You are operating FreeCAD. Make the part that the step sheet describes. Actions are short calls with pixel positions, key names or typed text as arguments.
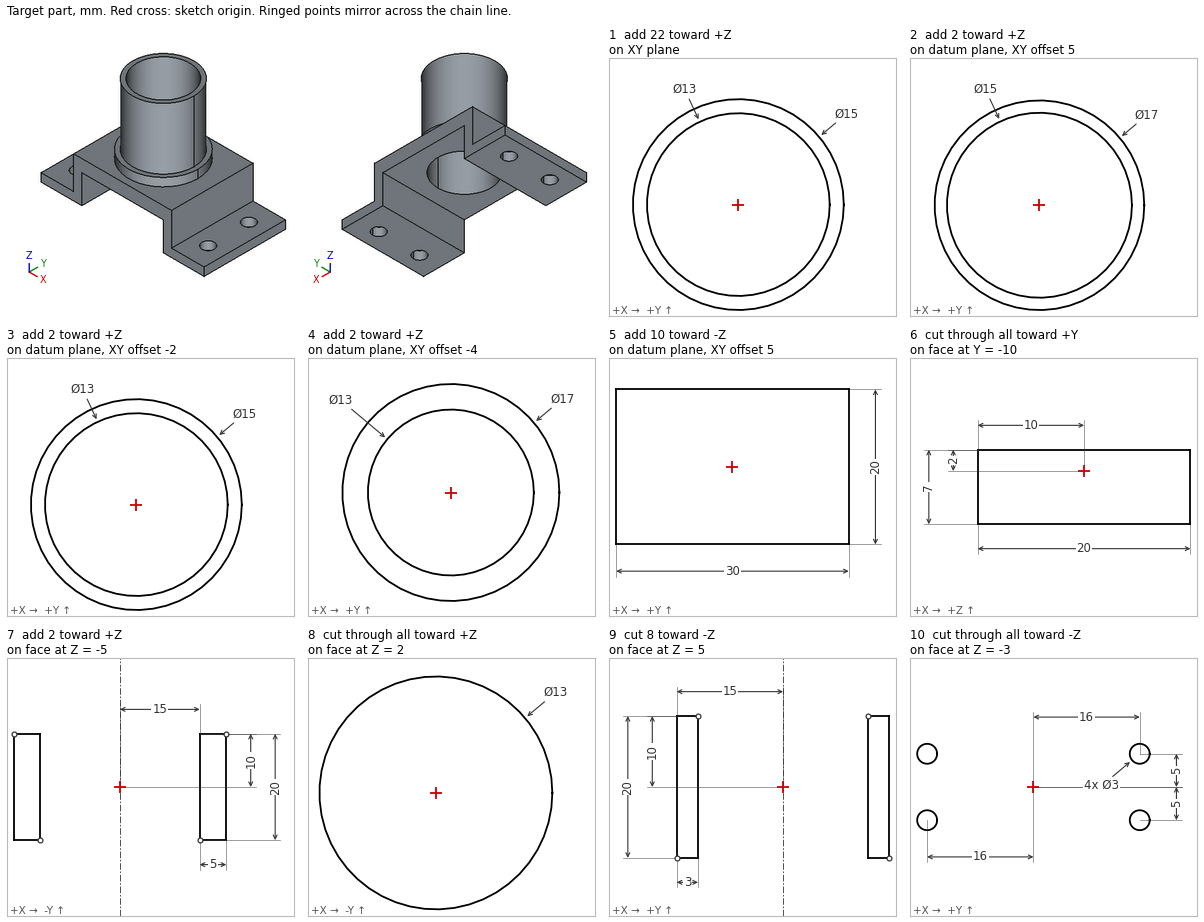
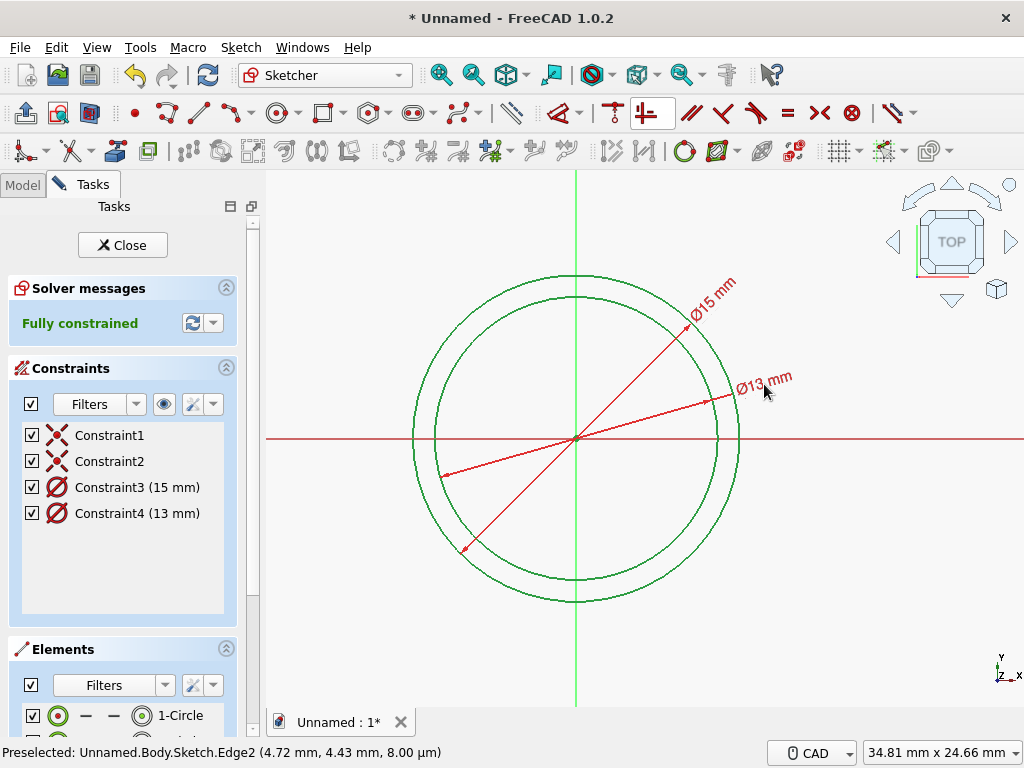
click(123, 245)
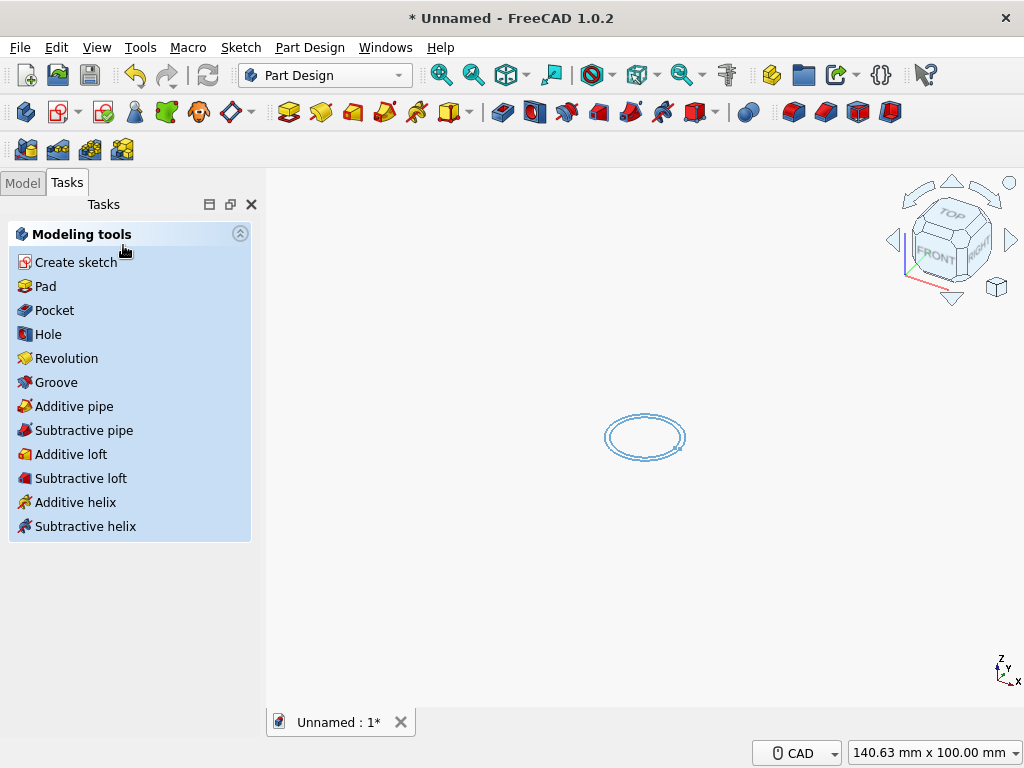
click(290, 112)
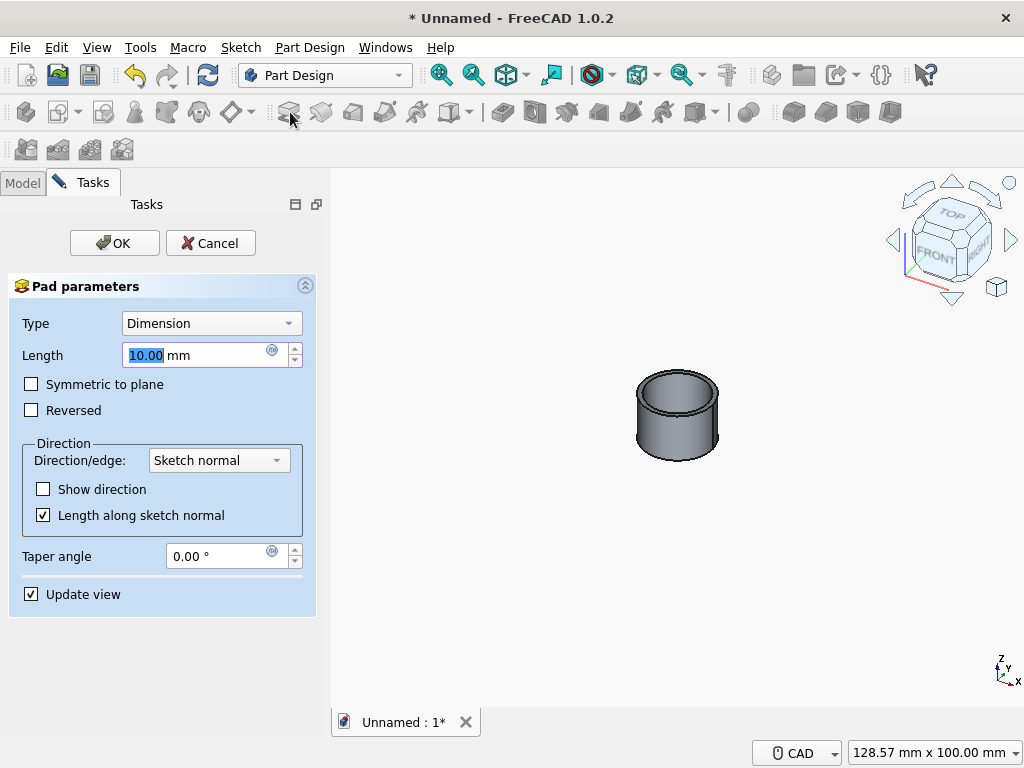
text(22)
key(Tab)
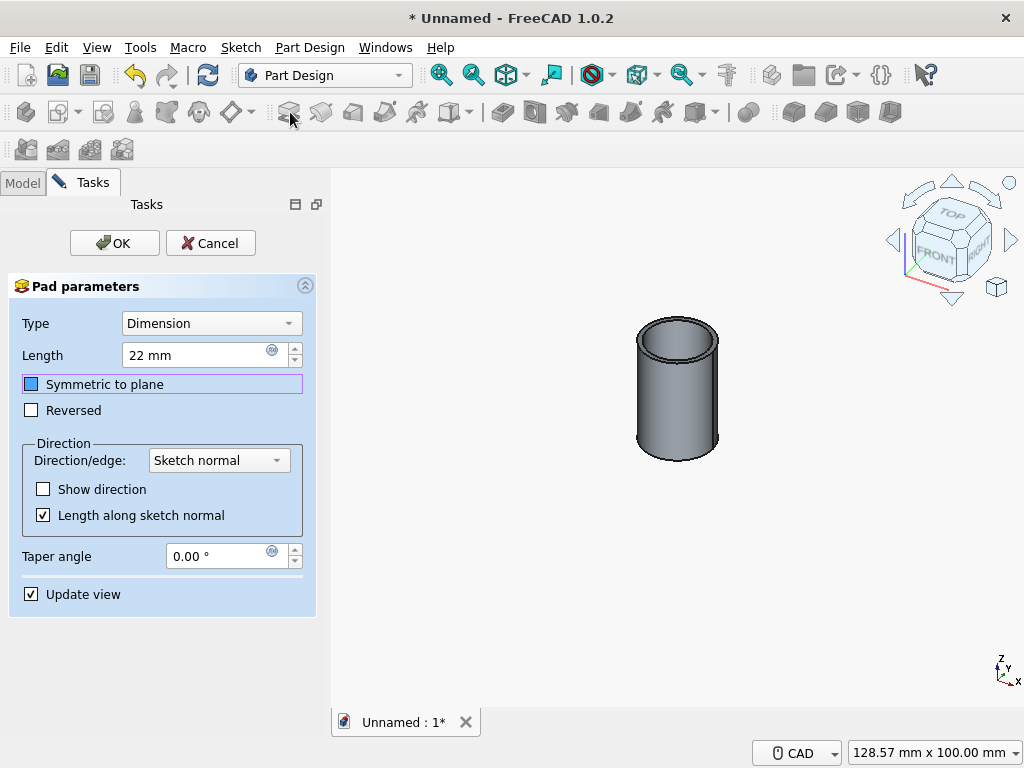
click(115, 243)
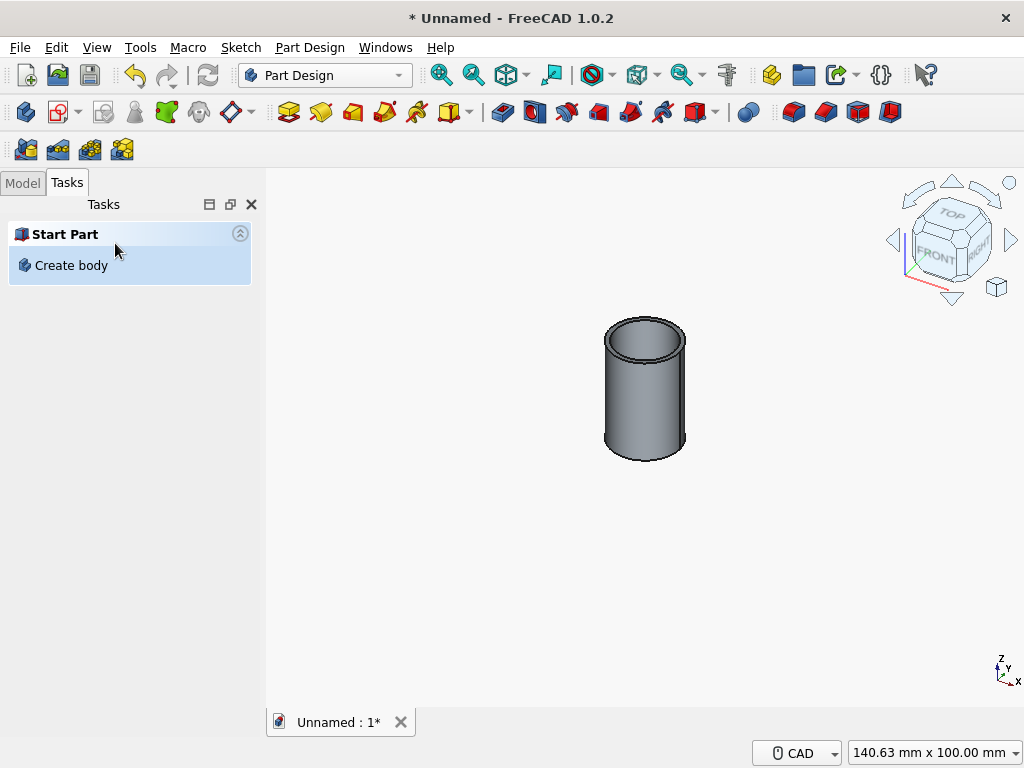
click(442, 76)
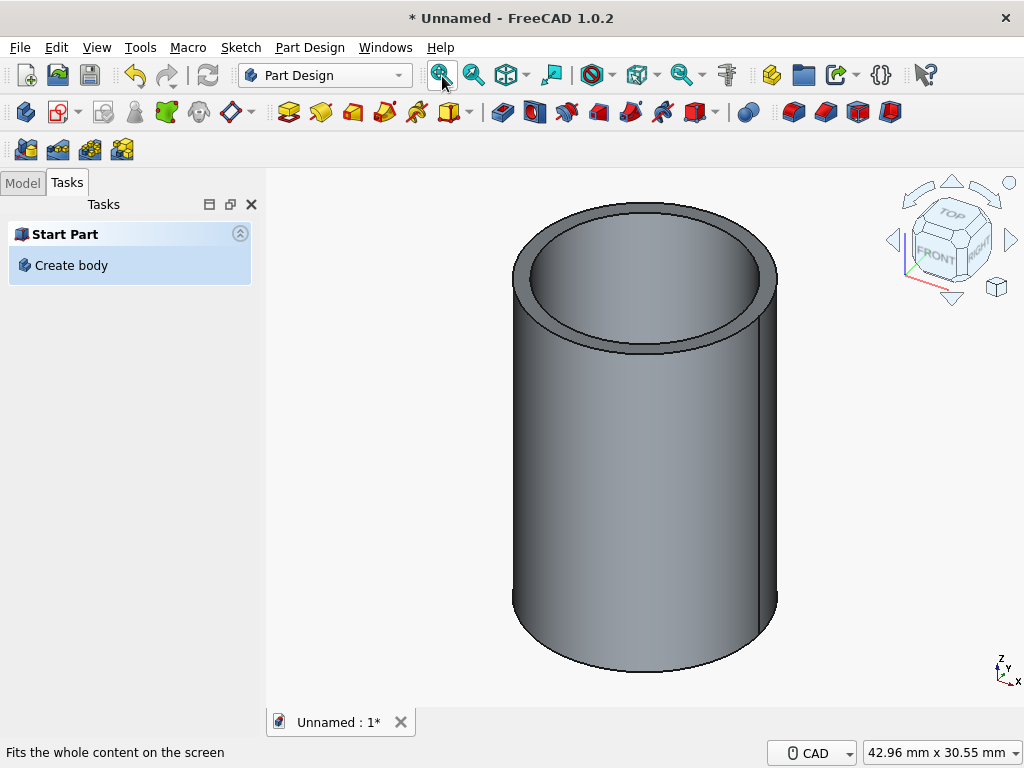
click(23, 182)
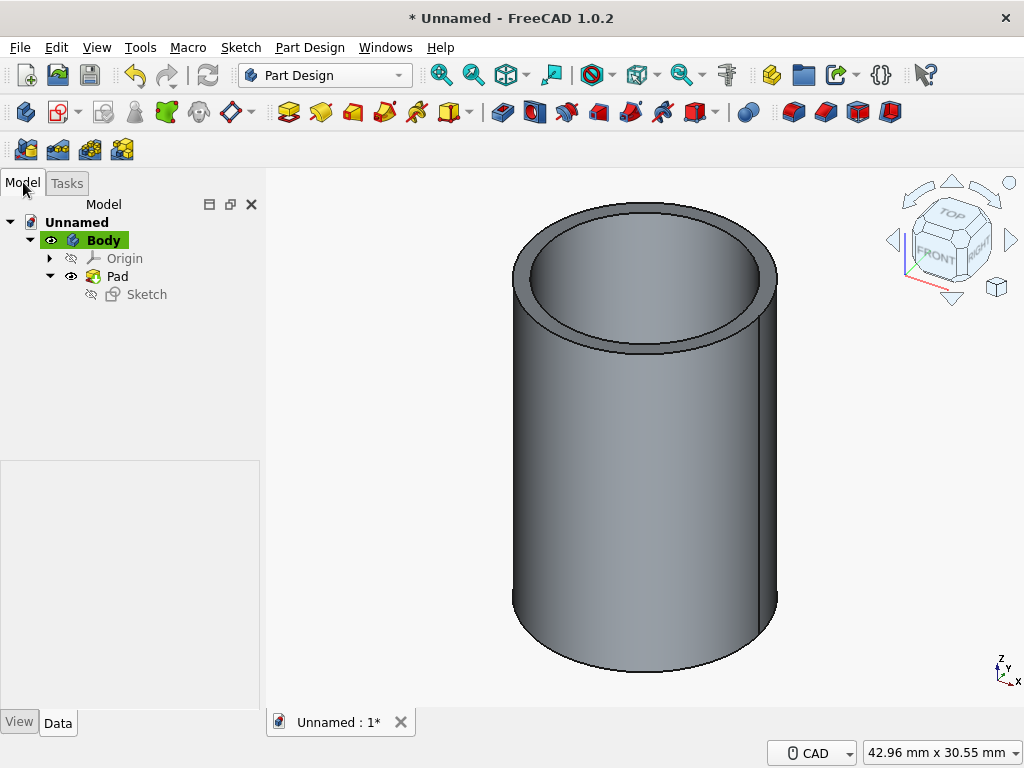
click(50, 258)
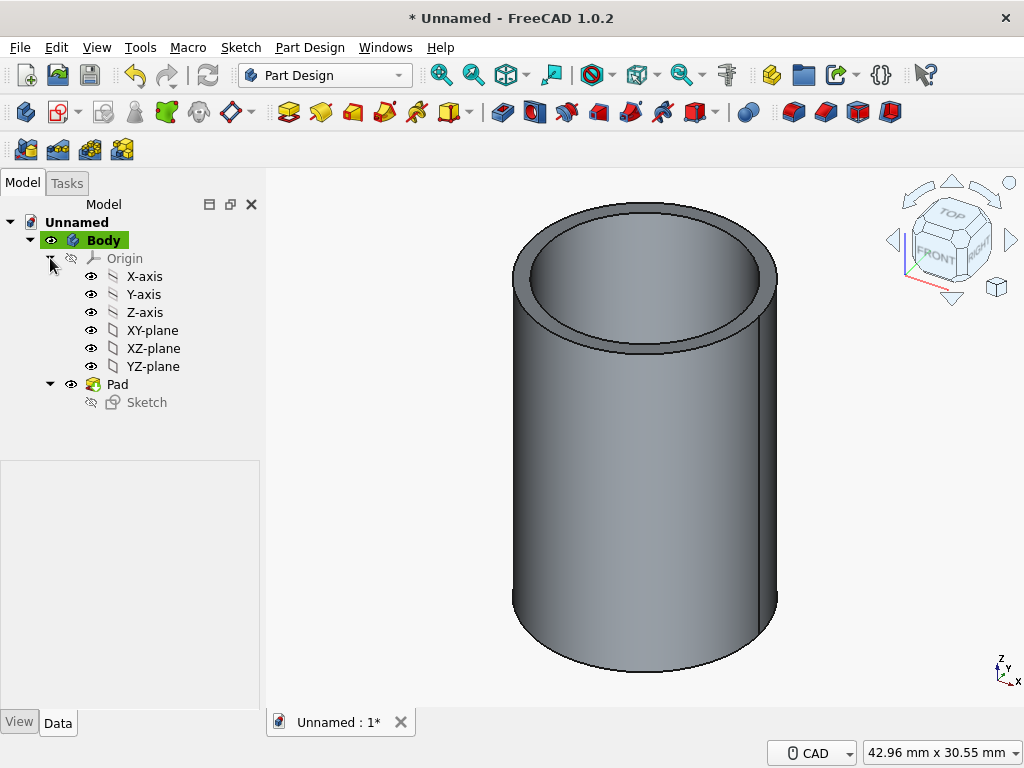
click(136, 330)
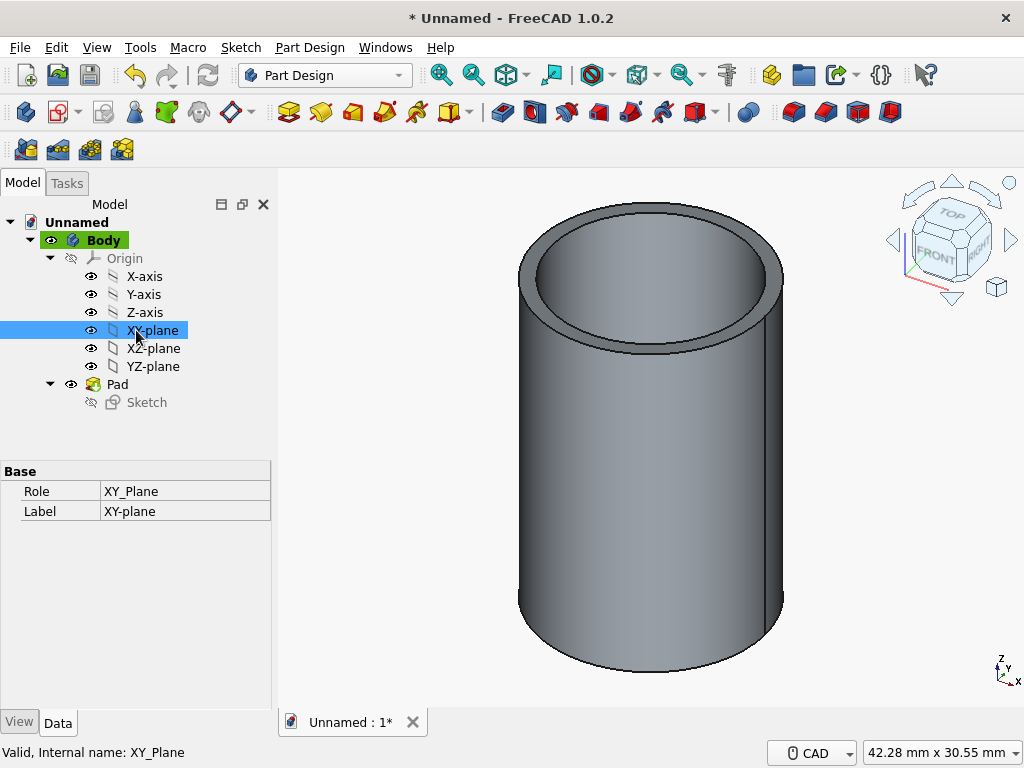
click(232, 112)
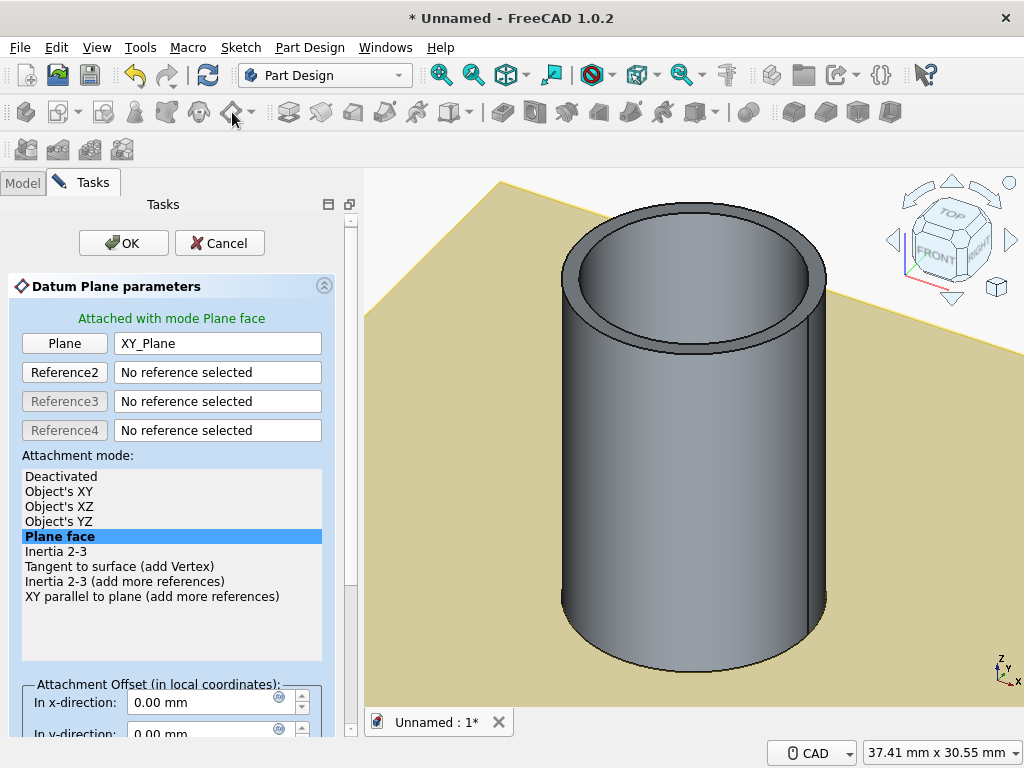
scroll(351, 475, down, 2)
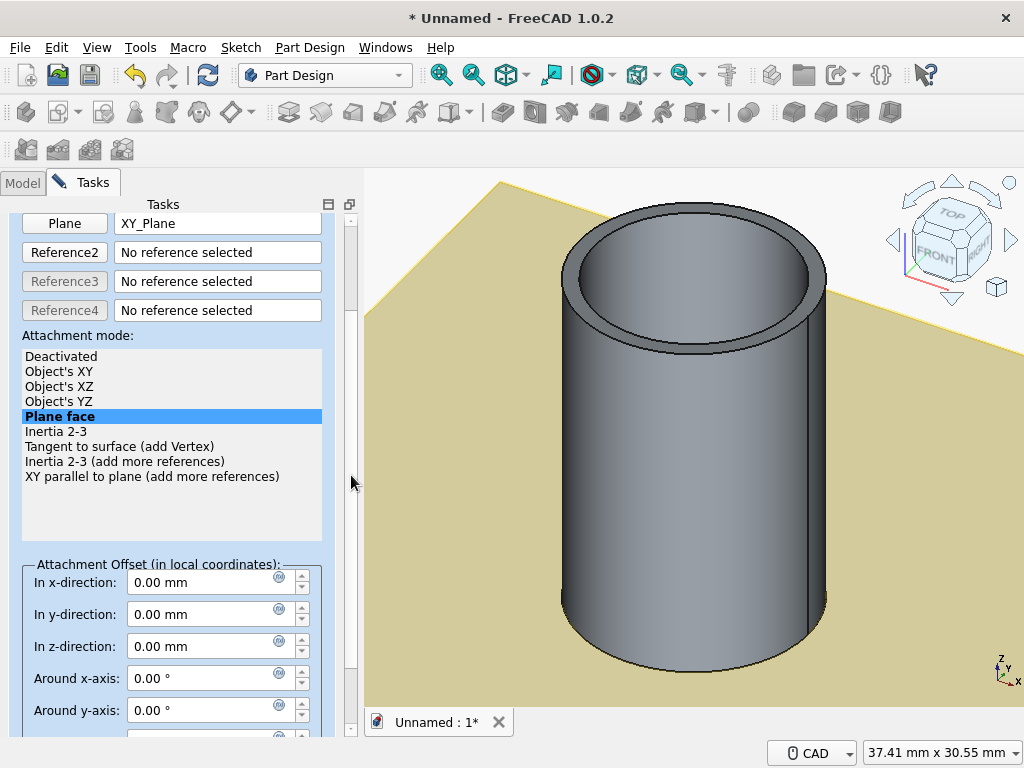
triple_click(210, 646)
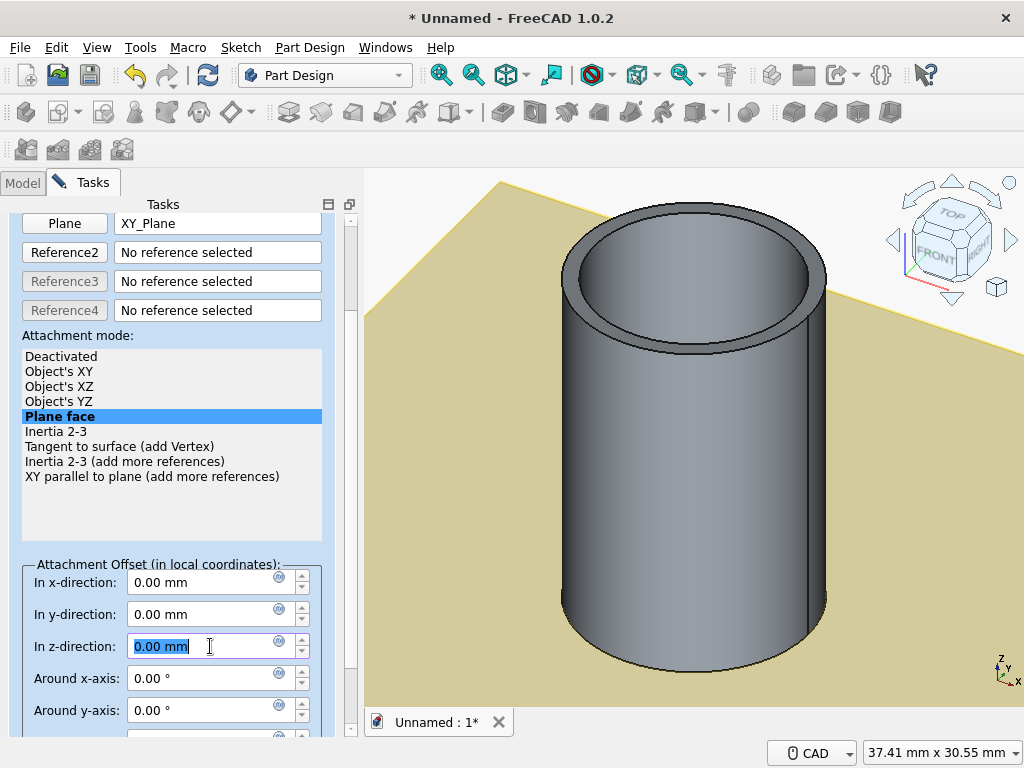
text(5)
key(Tab)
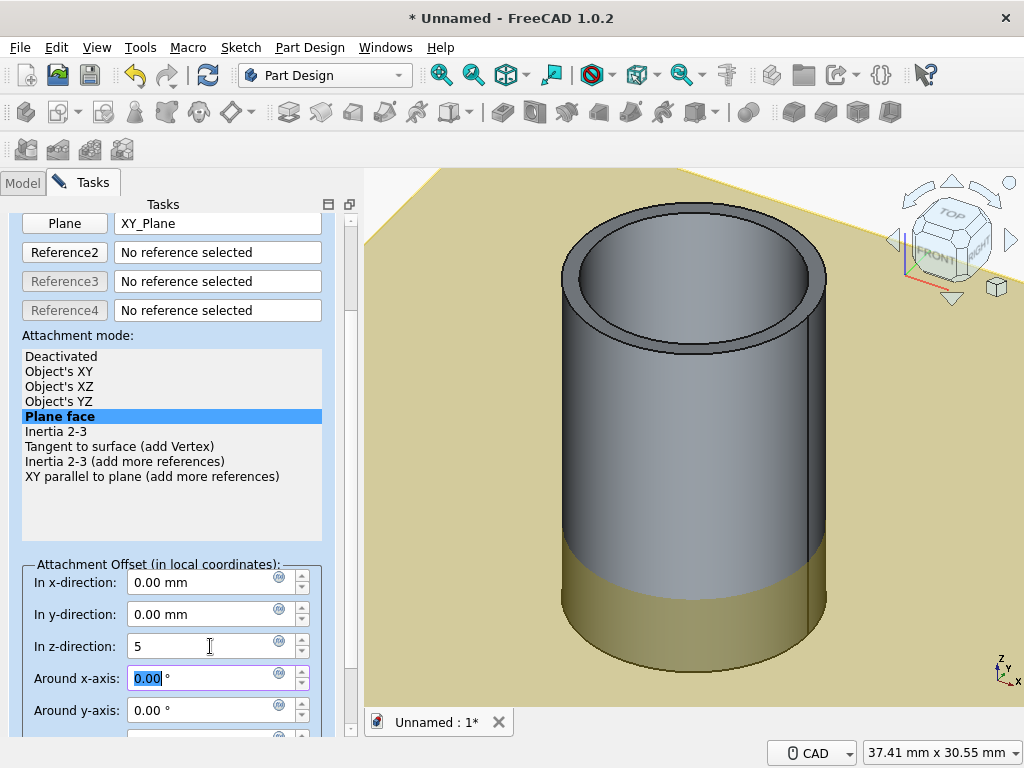
scroll(351, 475, up, 3)